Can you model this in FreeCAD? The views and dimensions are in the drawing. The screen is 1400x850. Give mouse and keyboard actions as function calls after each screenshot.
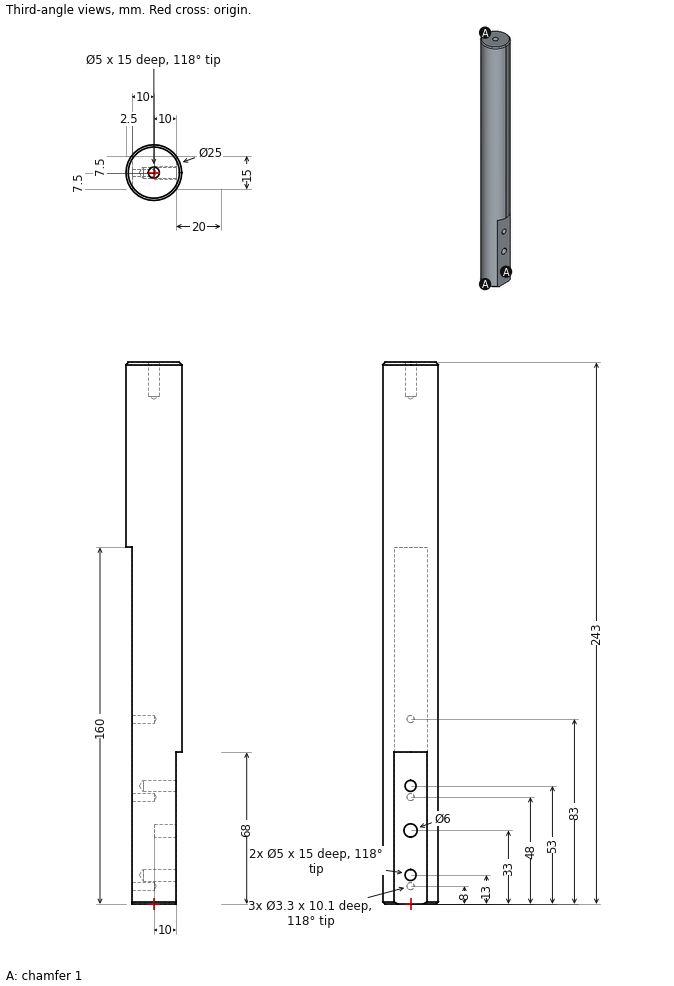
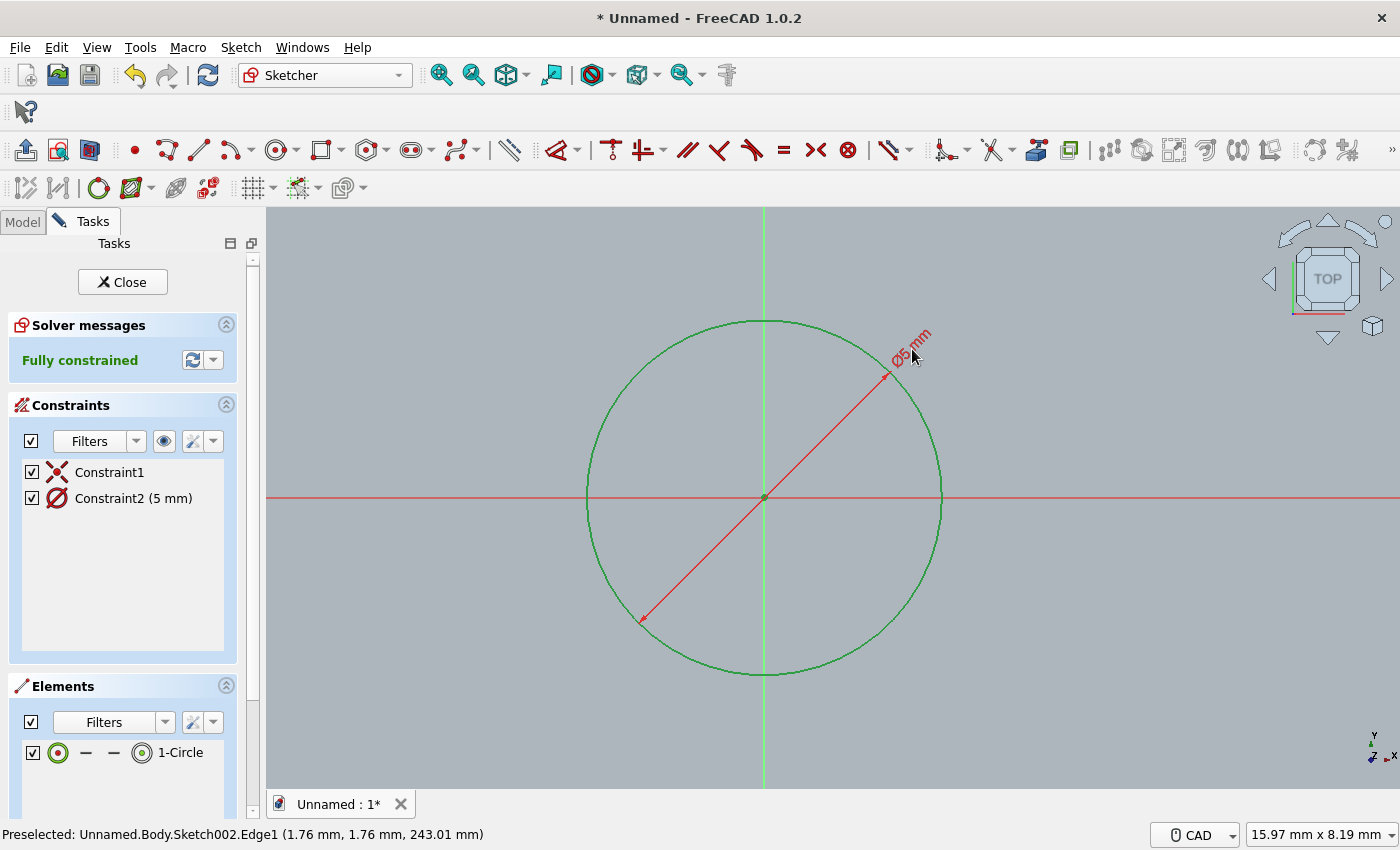
click(123, 282)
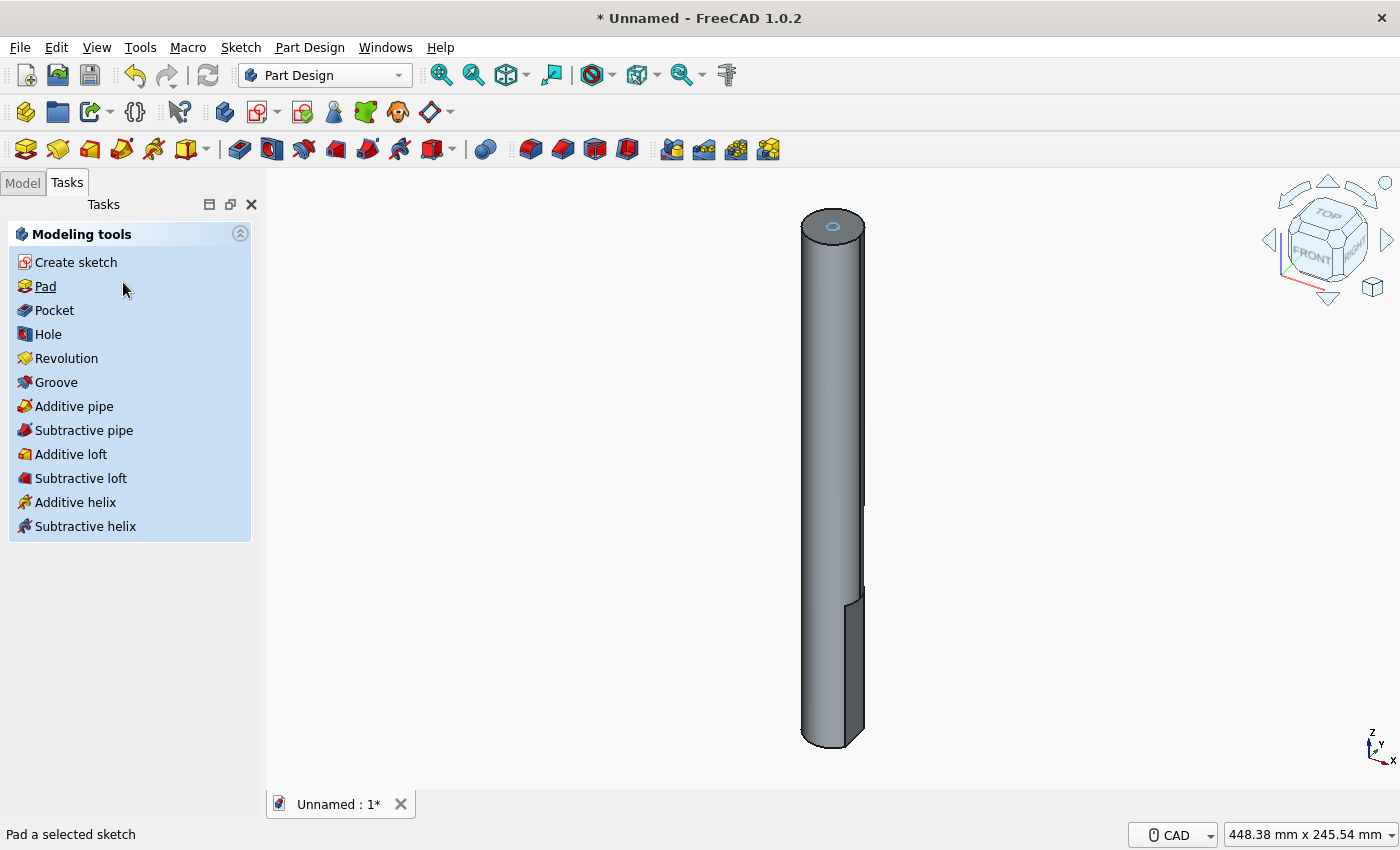
click(272, 150)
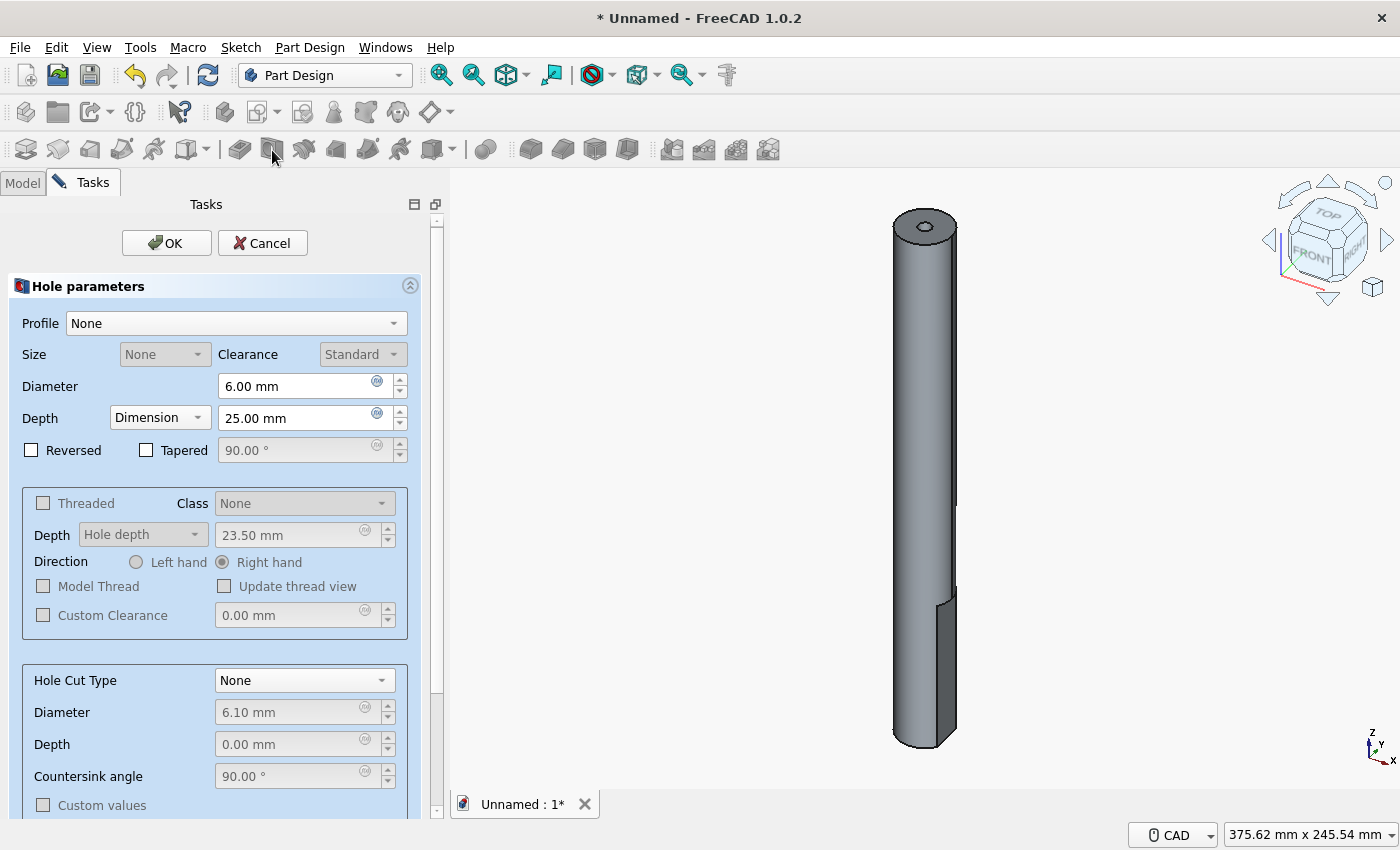
triple_click(305, 386)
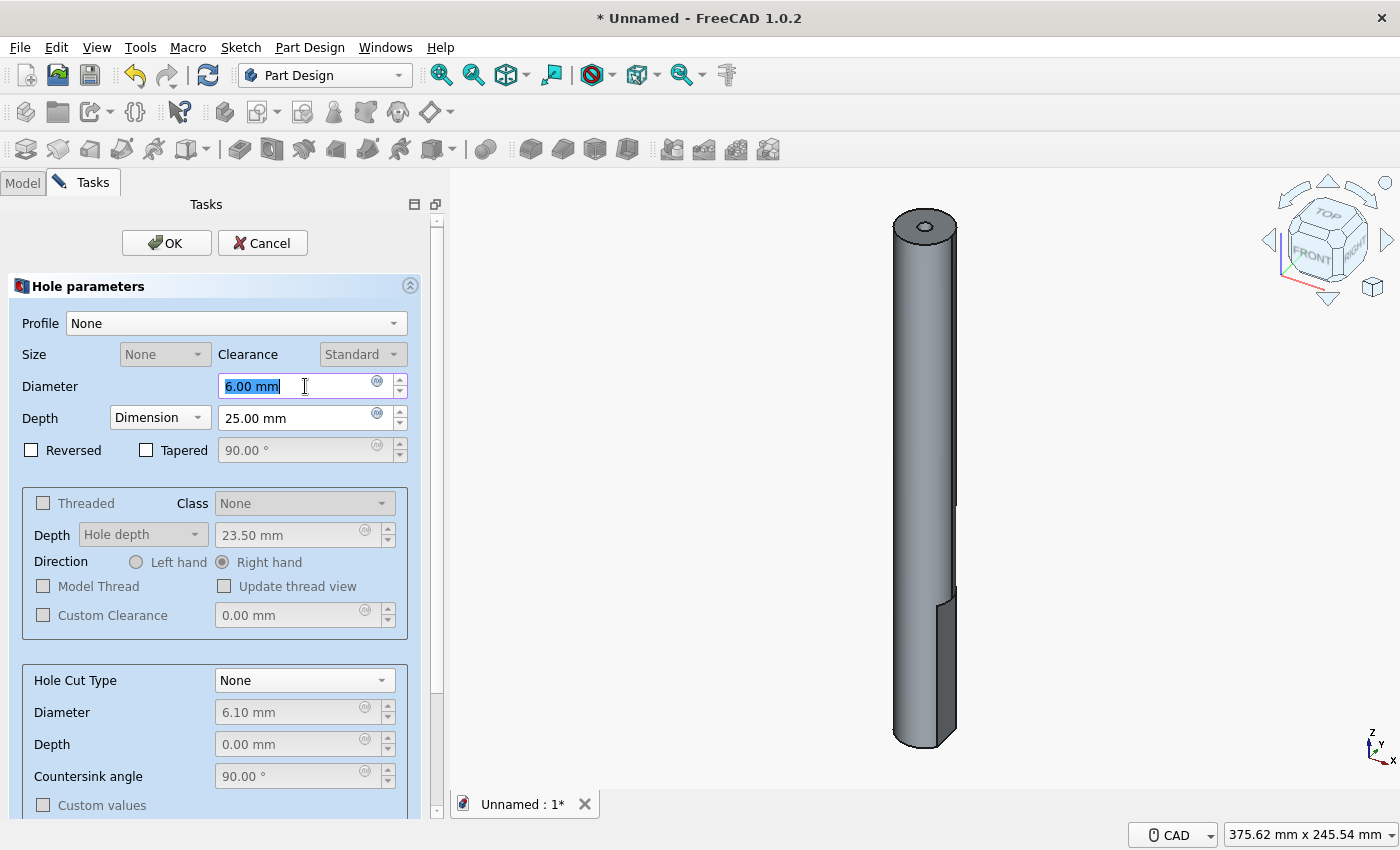
text(5)
key(Tab)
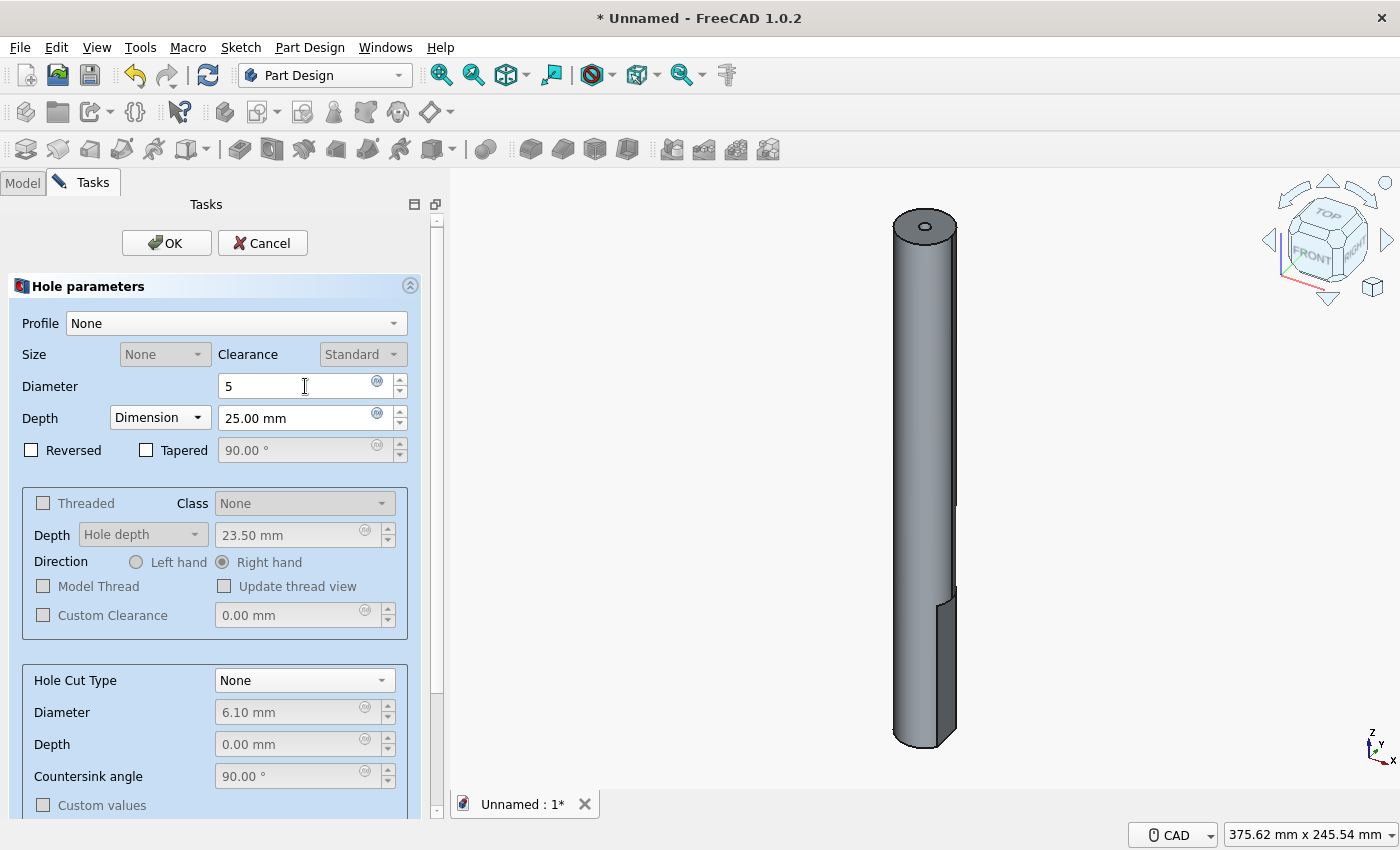
triple_click(305, 418)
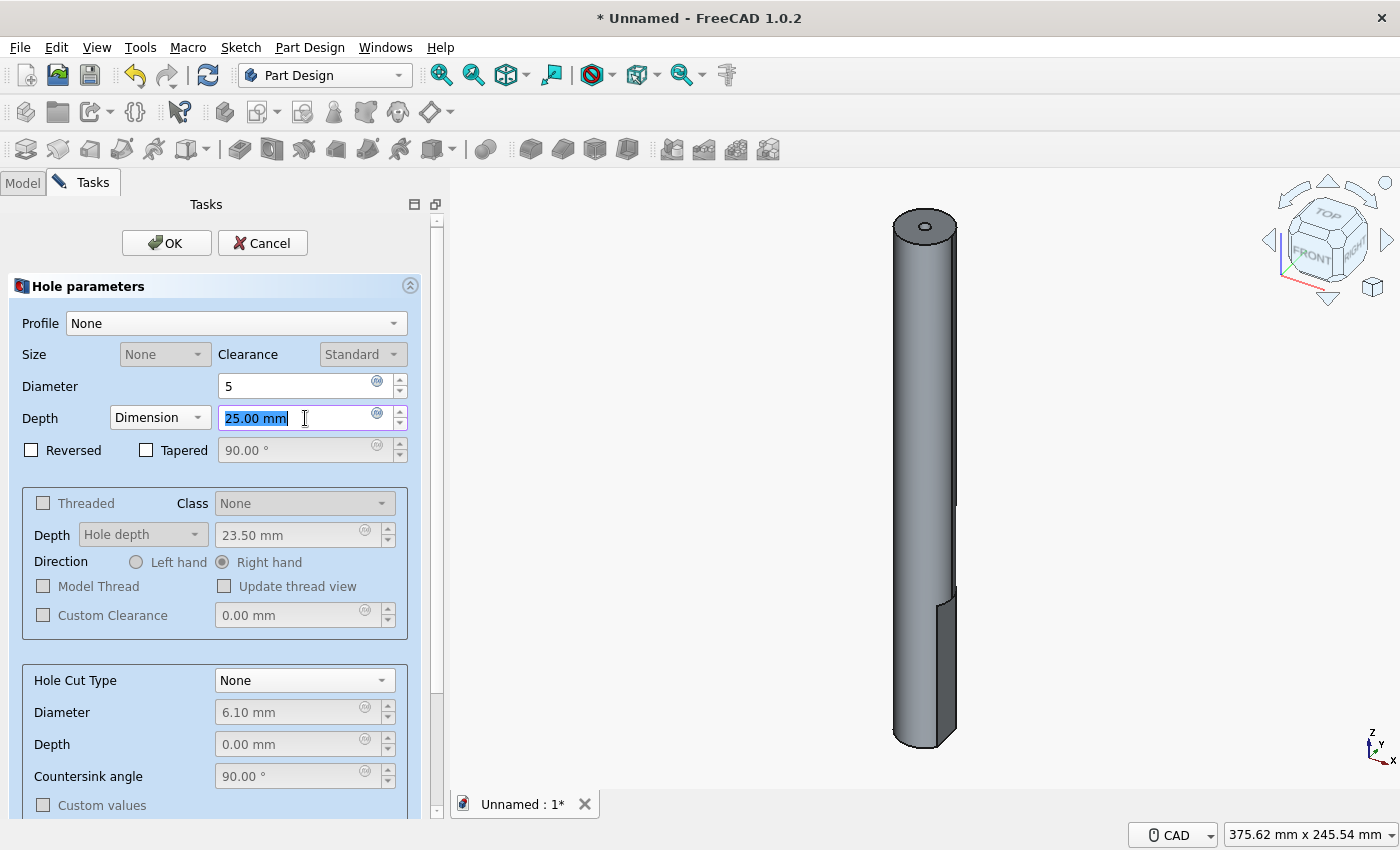
text(15)
key(Tab)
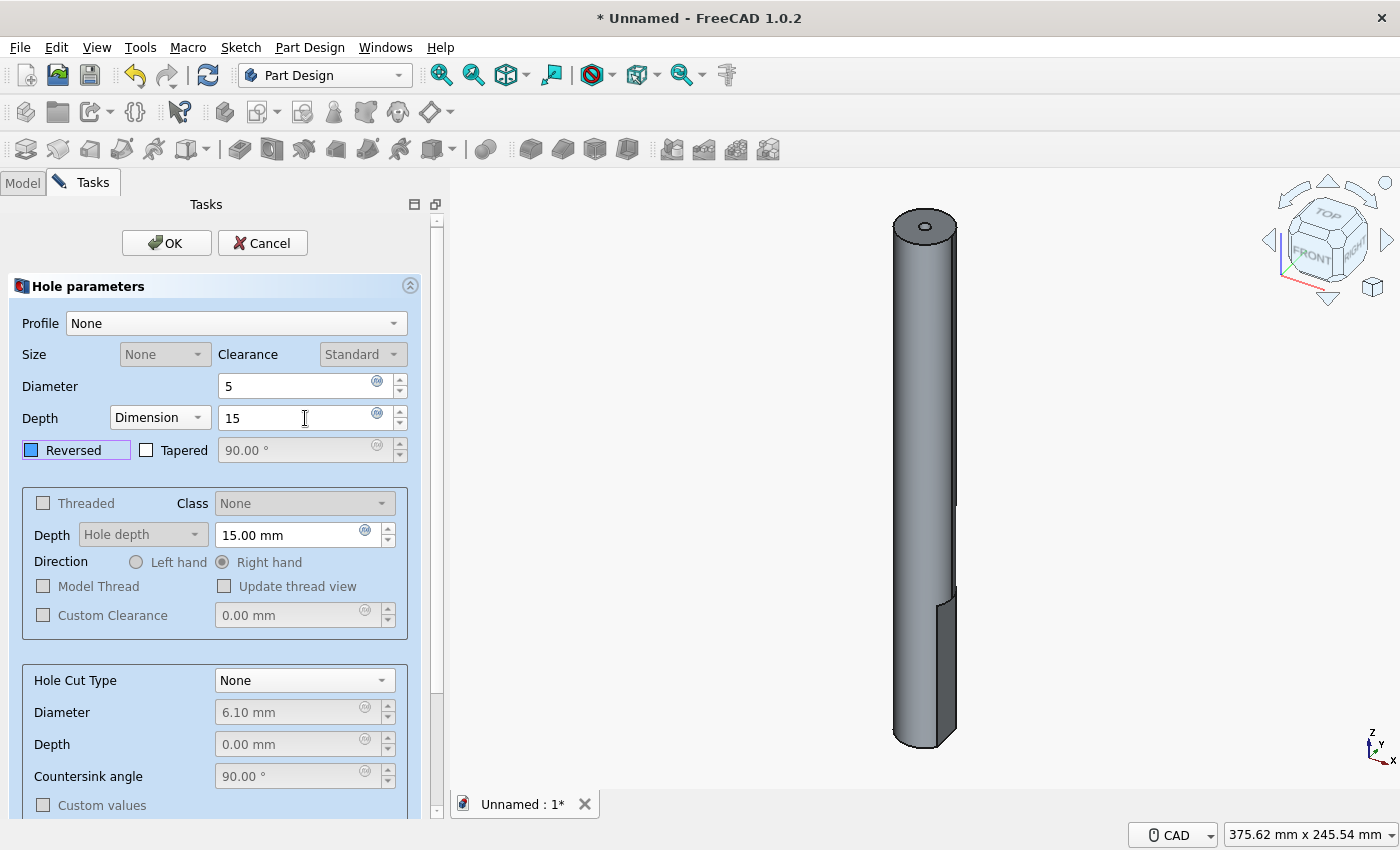
click(167, 243)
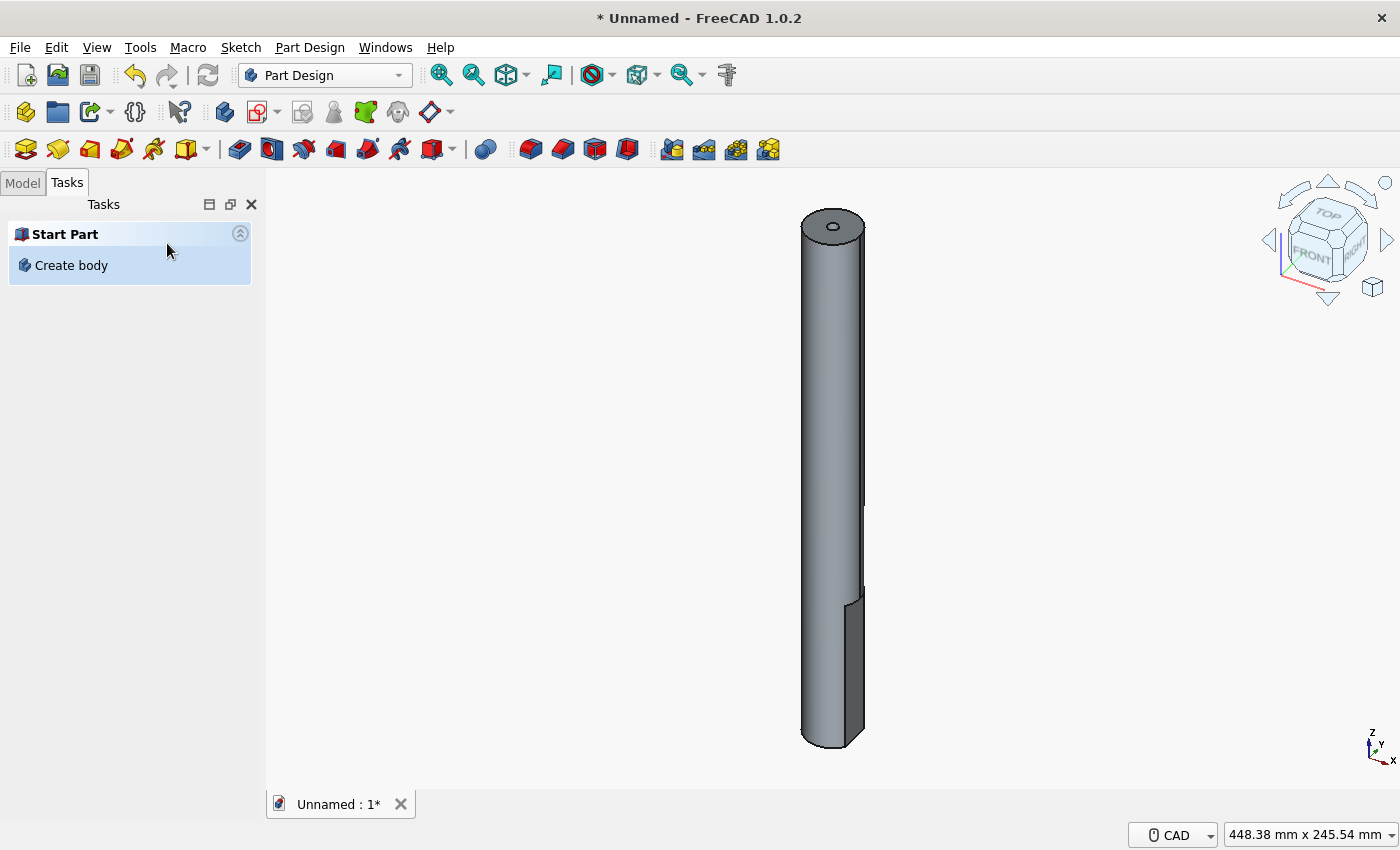
click(855, 626)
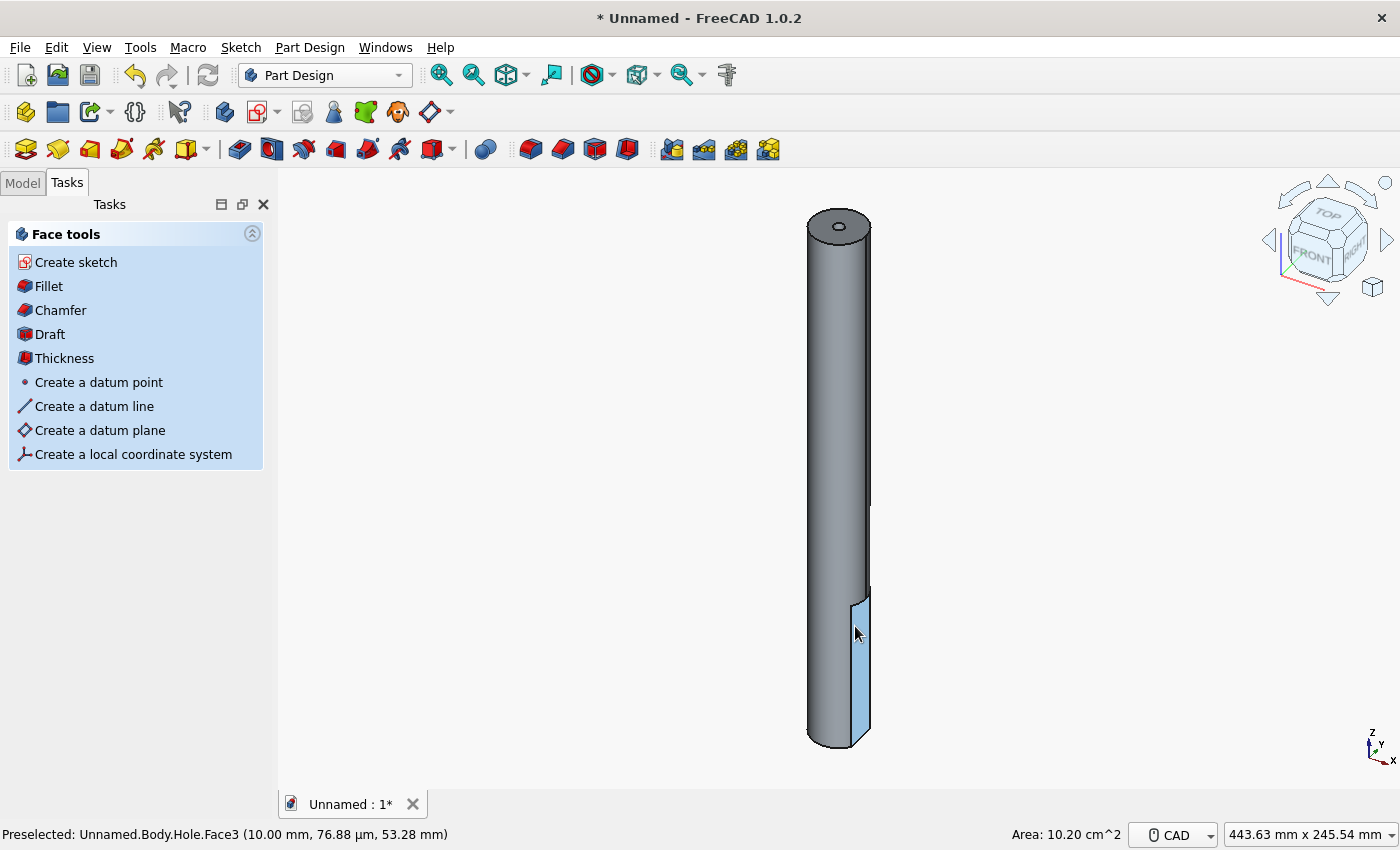
click(258, 112)